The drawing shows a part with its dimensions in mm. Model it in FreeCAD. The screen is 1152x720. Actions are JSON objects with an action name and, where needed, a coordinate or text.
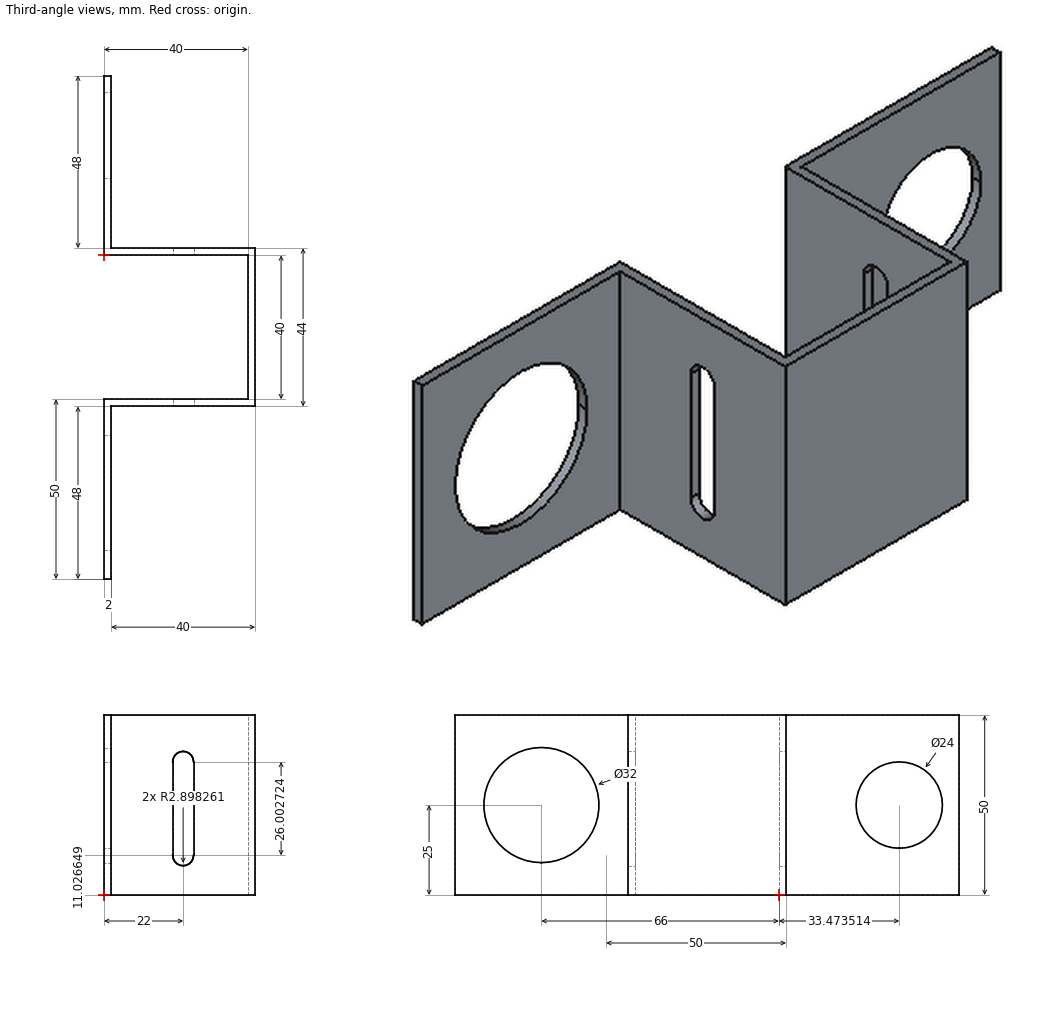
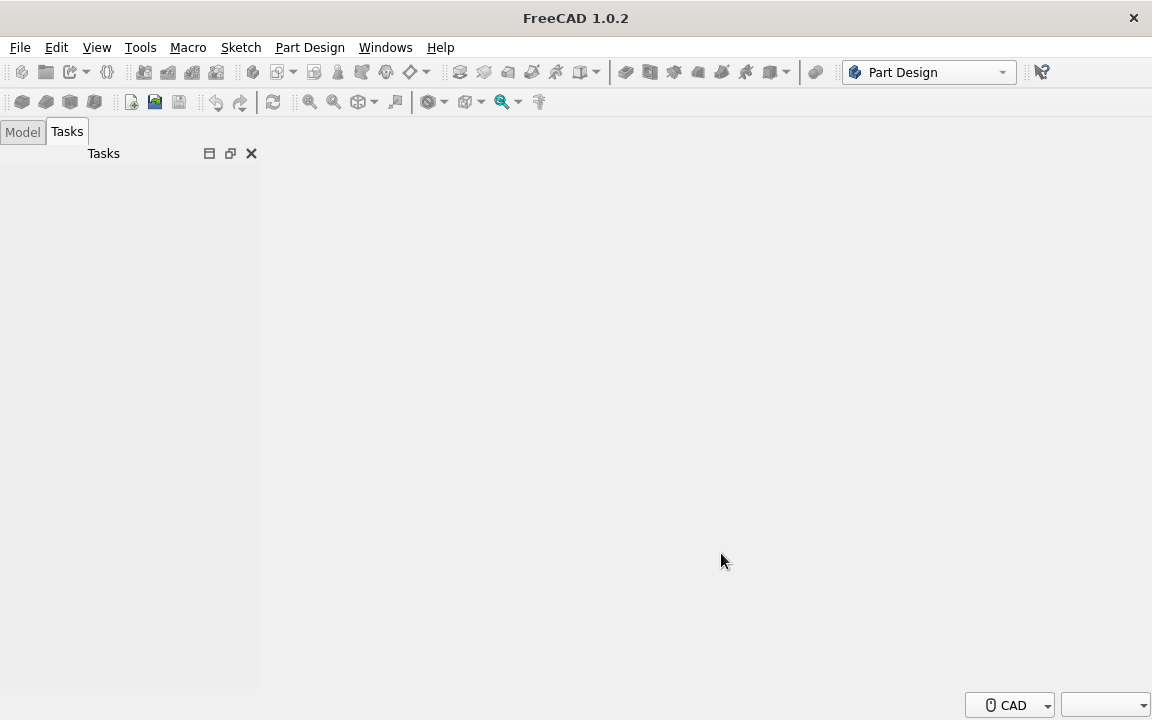
{"action": "left_click", "coordinate": [132, 102]}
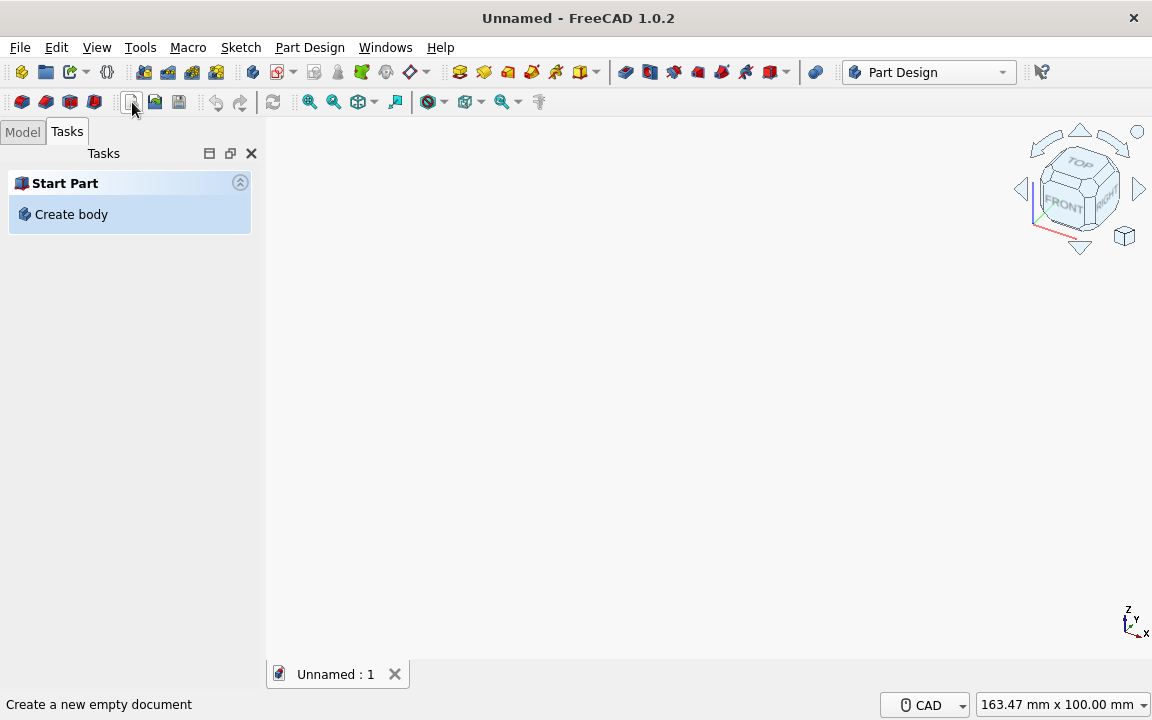
{"action": "left_click", "coordinate": [278, 72]}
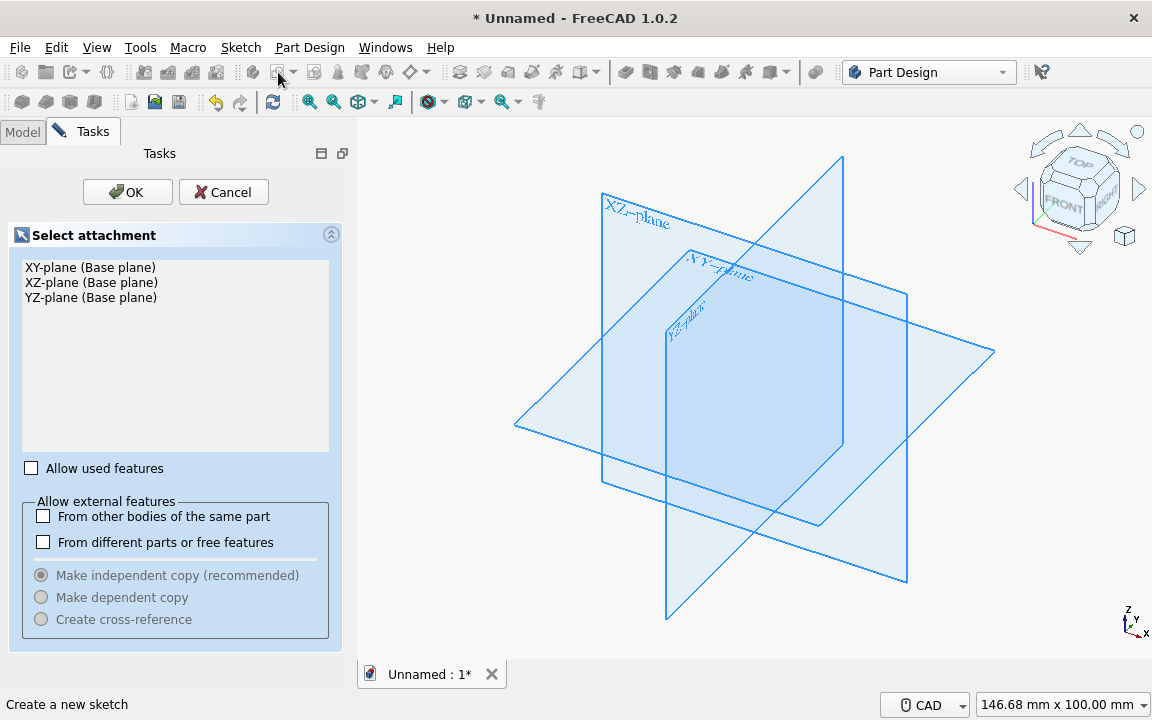
{"action": "left_click", "coordinate": [82, 268]}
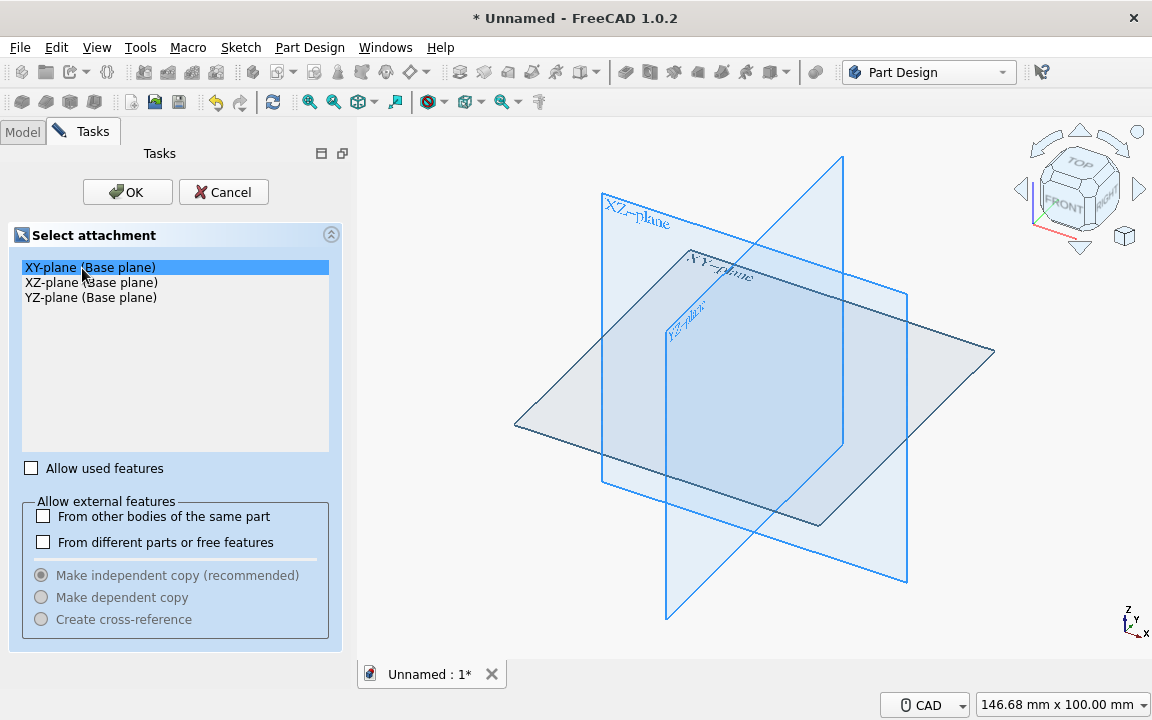
{"action": "left_click", "coordinate": [128, 192]}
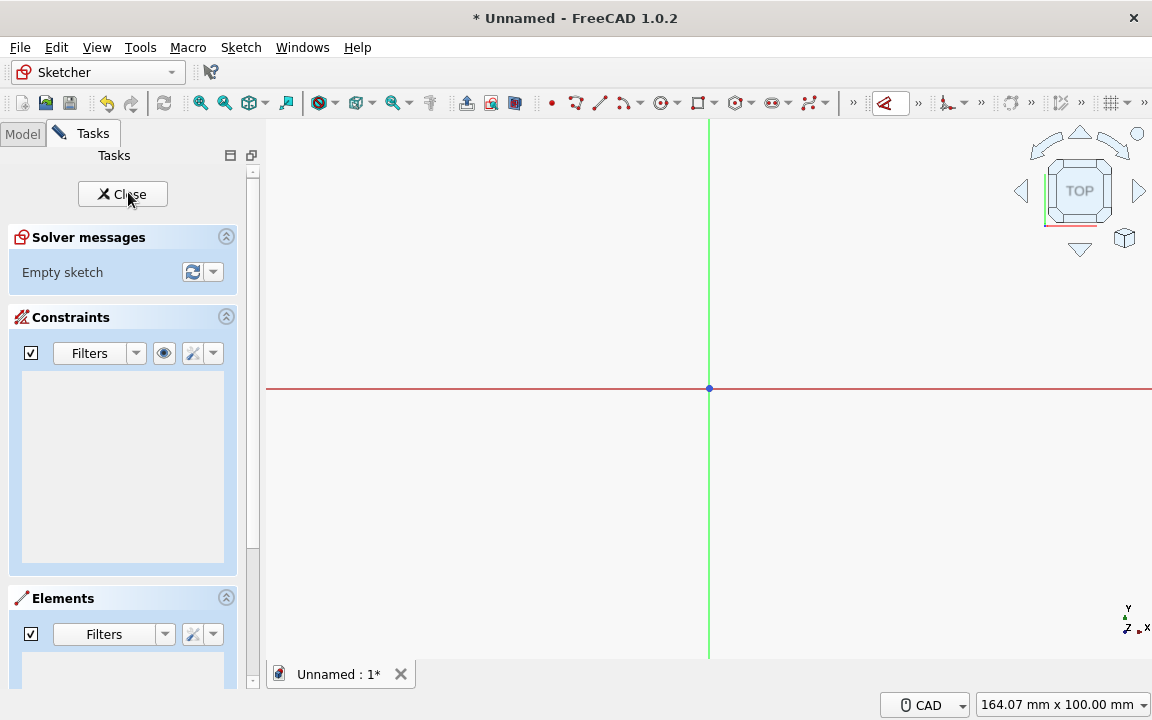
{"action": "scroll", "coordinate": [492, 301], "scroll_direction": "down", "scroll_amount": 4}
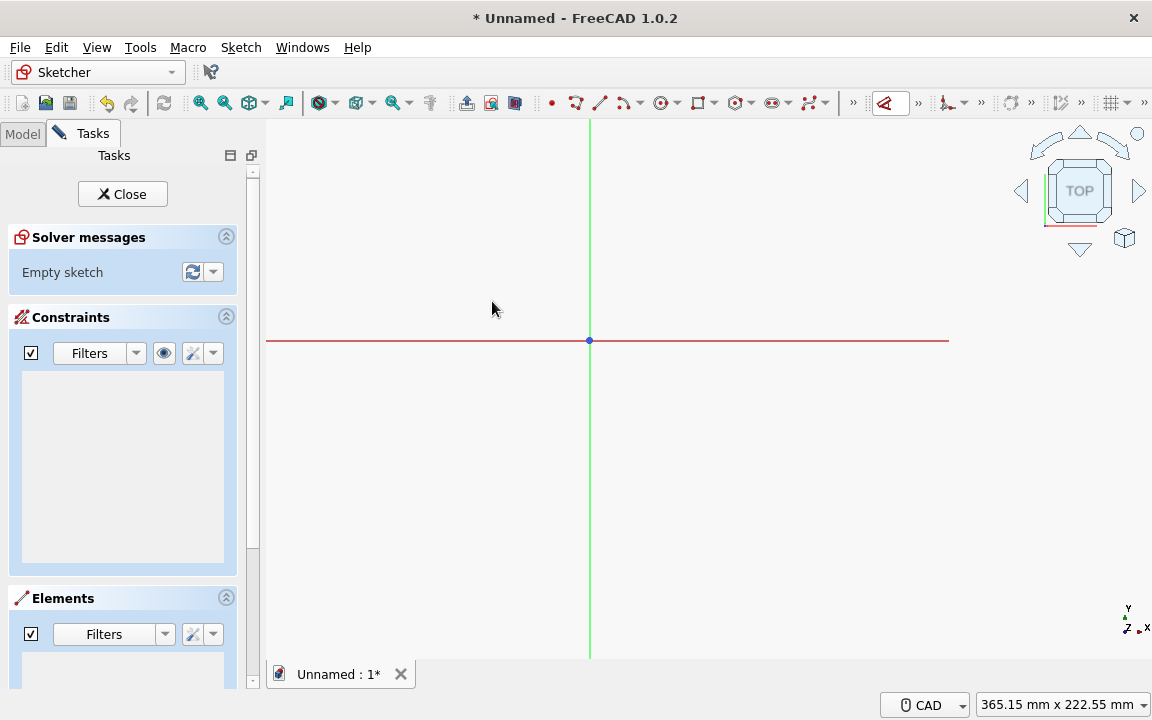
{"action": "key", "text": "g m"}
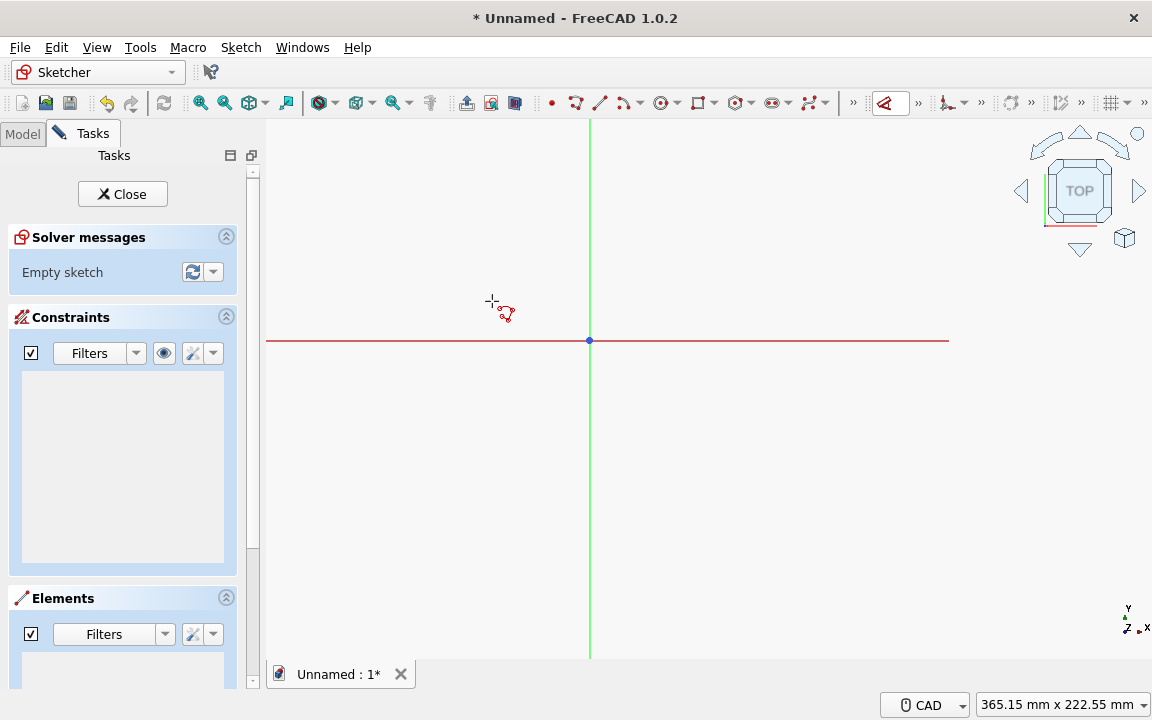
{"action": "left_click", "coordinate": [590, 341]}
{"action": "left_click", "coordinate": [687, 350]}
{"action": "left_click", "coordinate": [687, 438]}
{"action": "left_click", "coordinate": [590, 438]}
{"action": "left_click", "coordinate": [599, 559]}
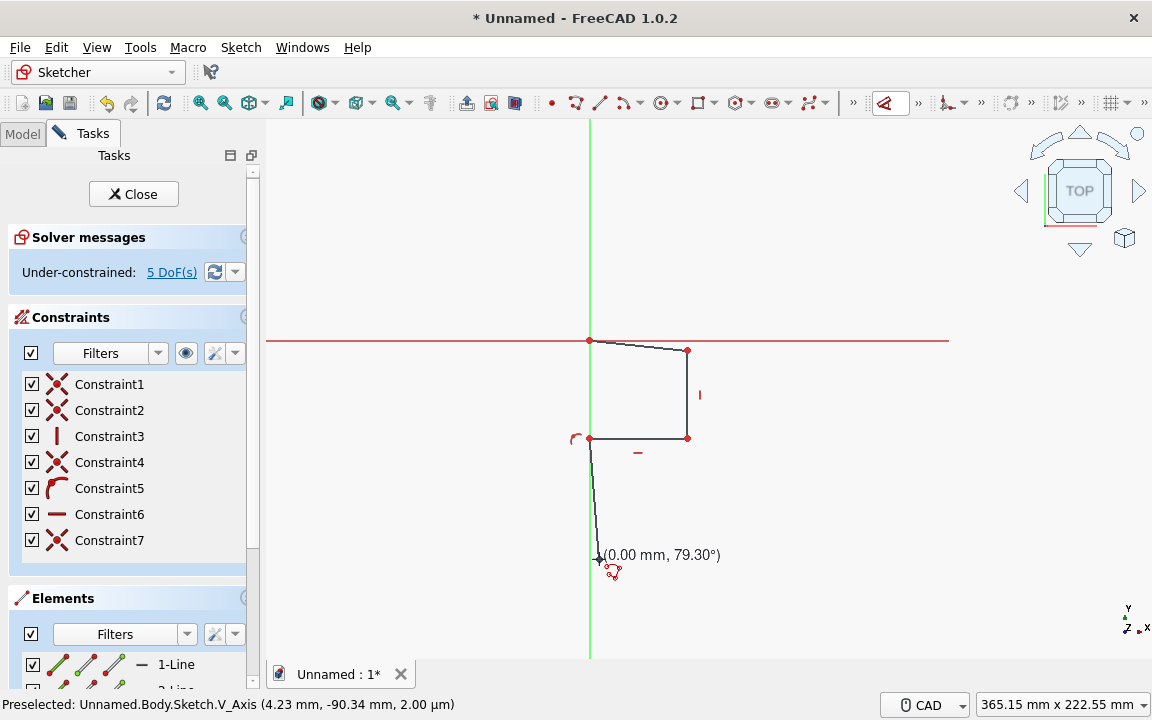
{"action": "scroll", "coordinate": [594, 559], "scroll_direction": "up", "scroll_amount": 6}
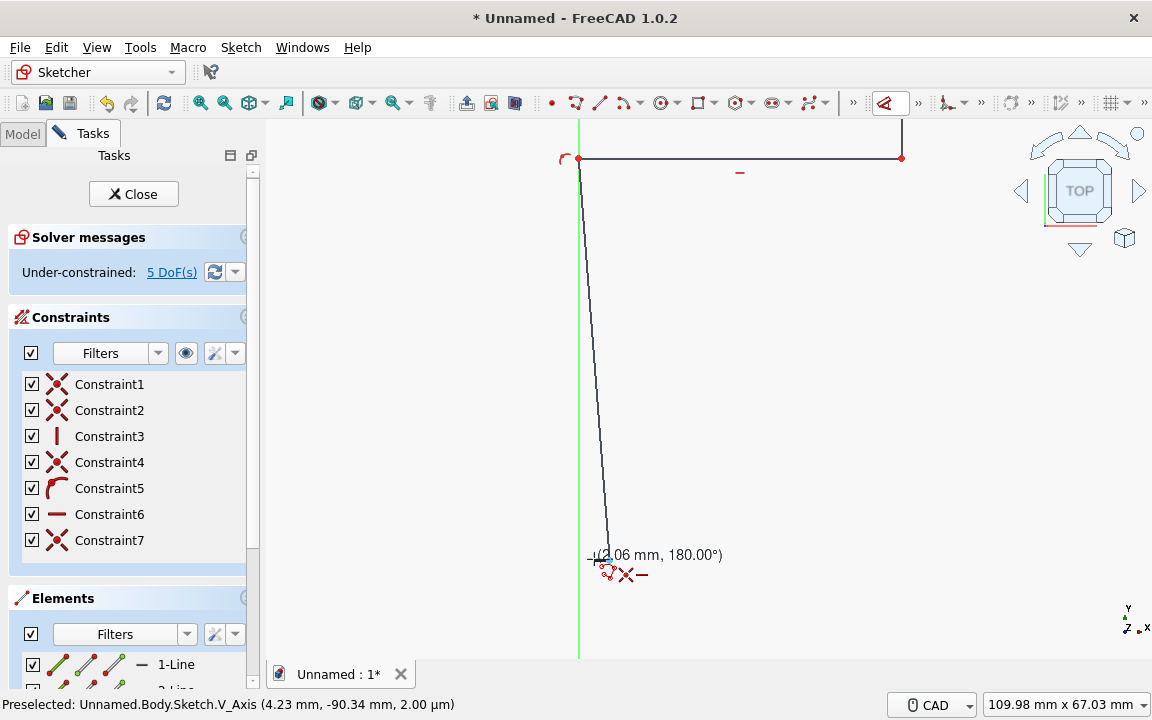
{"action": "left_click", "coordinate": [595, 557]}
{"action": "left_click", "coordinate": [595, 171]}
{"action": "left_click", "coordinate": [917, 171]}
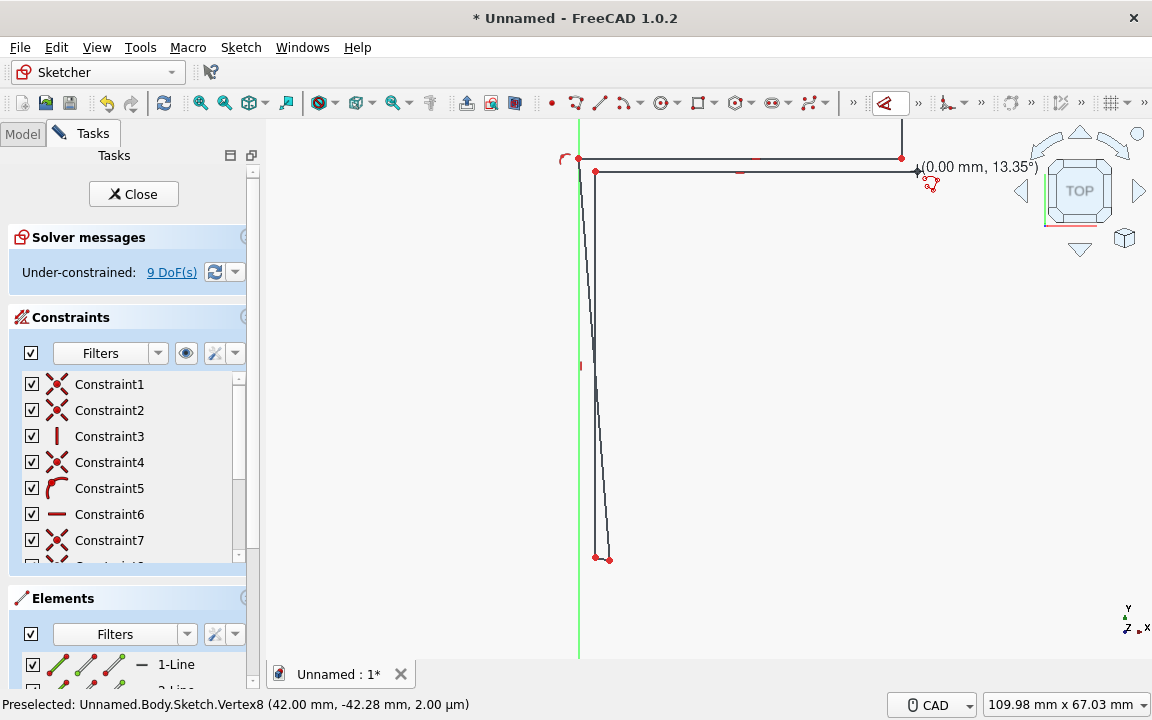
{"action": "scroll", "coordinate": [594, 559], "scroll_direction": "down", "scroll_amount": 6}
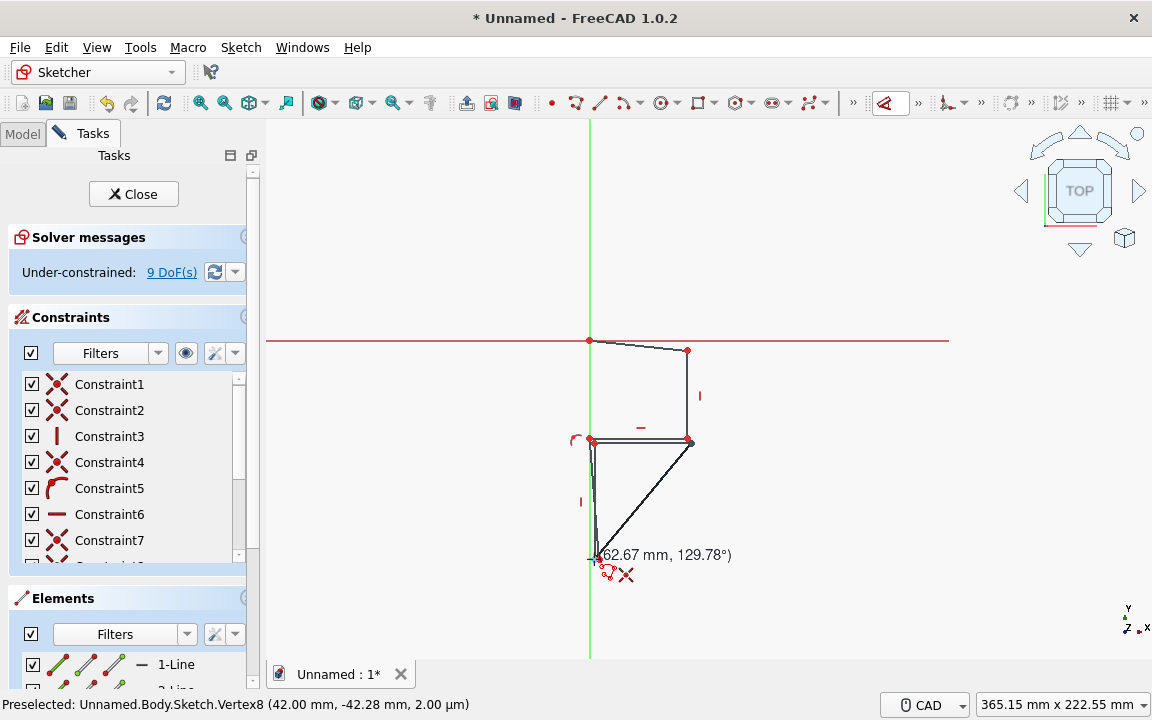
{"action": "scroll", "coordinate": [692, 336], "scroll_direction": "up", "scroll_amount": 6}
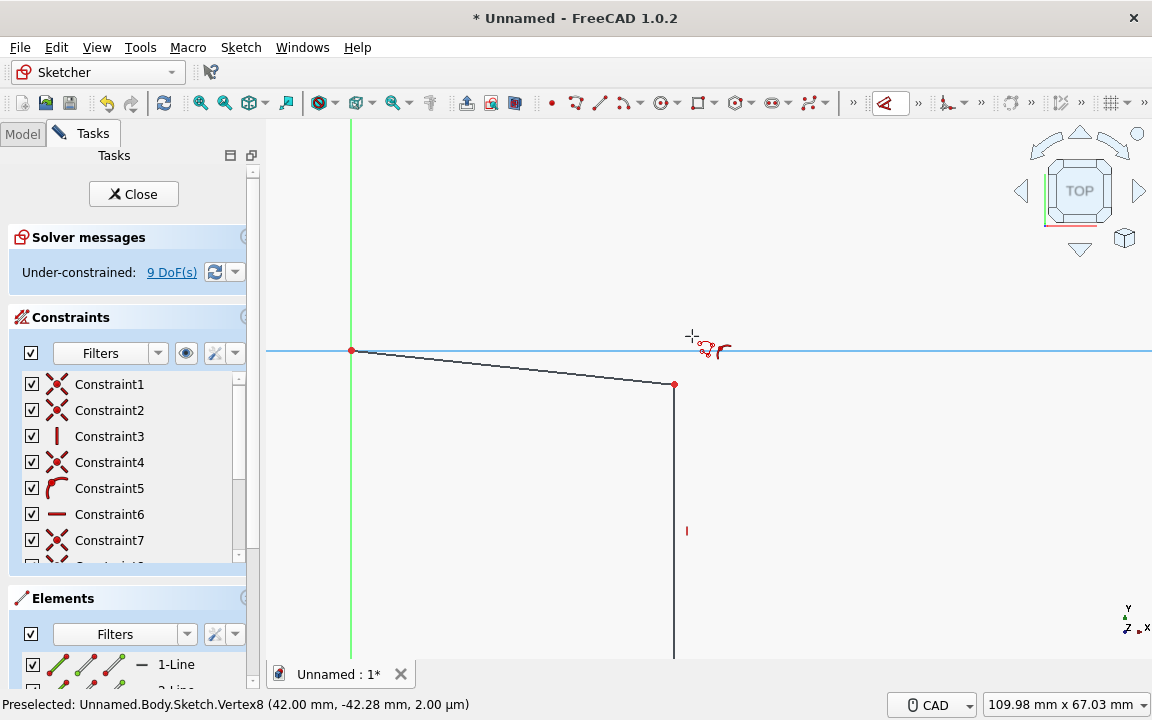
{"action": "left_click", "coordinate": [689, 335]}
{"action": "left_click", "coordinate": [367, 335]}